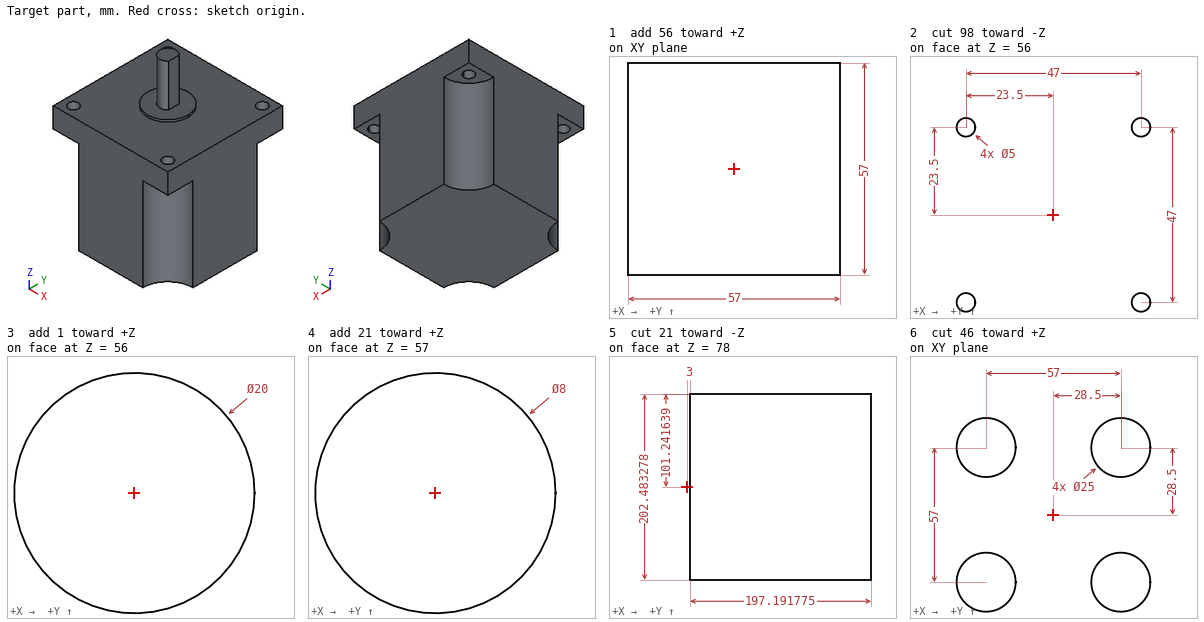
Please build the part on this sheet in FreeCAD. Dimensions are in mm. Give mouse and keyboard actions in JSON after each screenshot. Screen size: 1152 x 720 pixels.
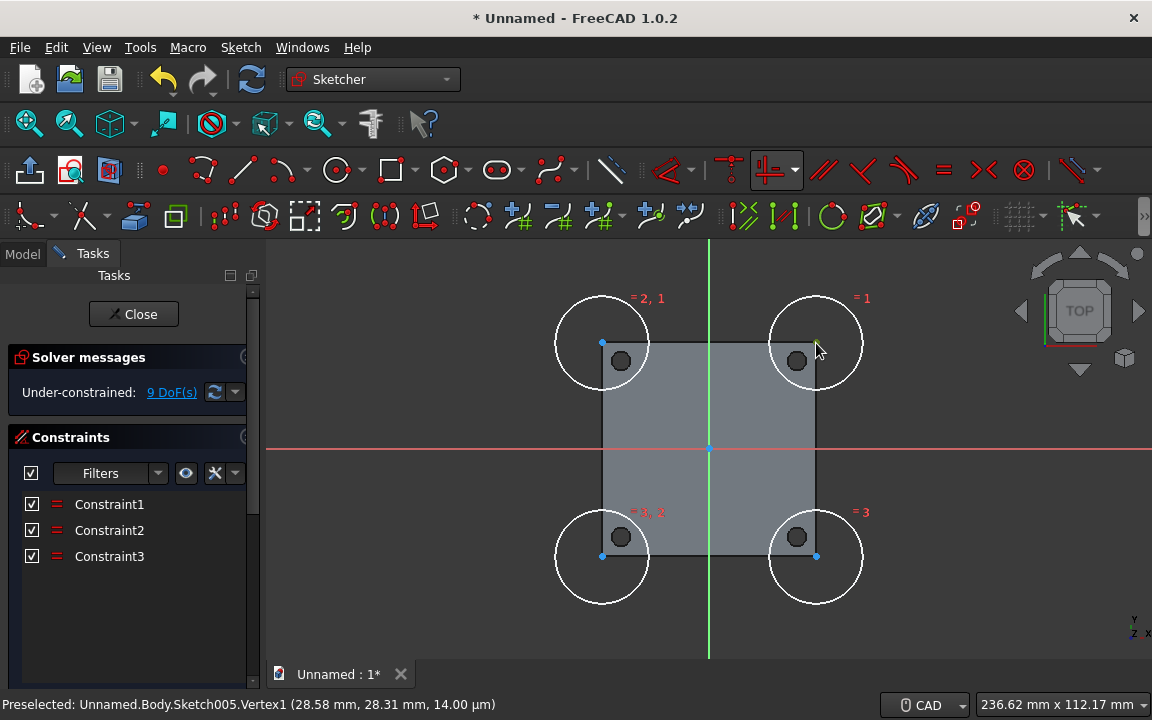
{"action": "left_click", "coordinate": [602, 343]}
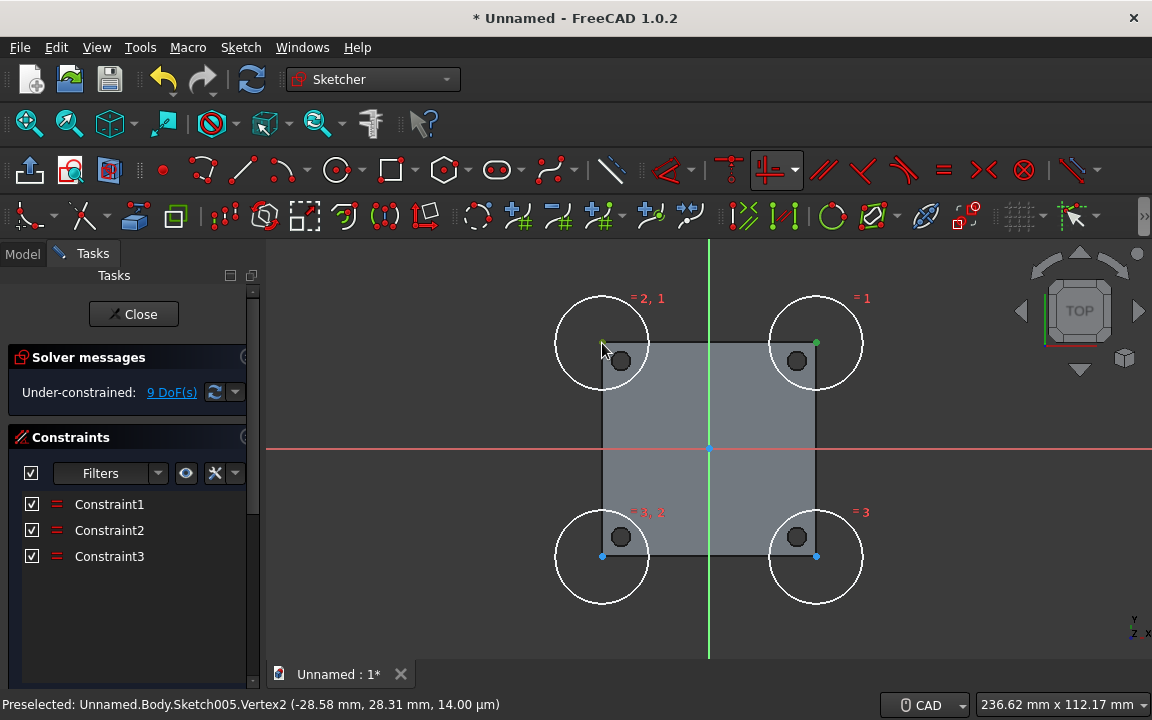
{"action": "left_click", "coordinate": [798, 170]}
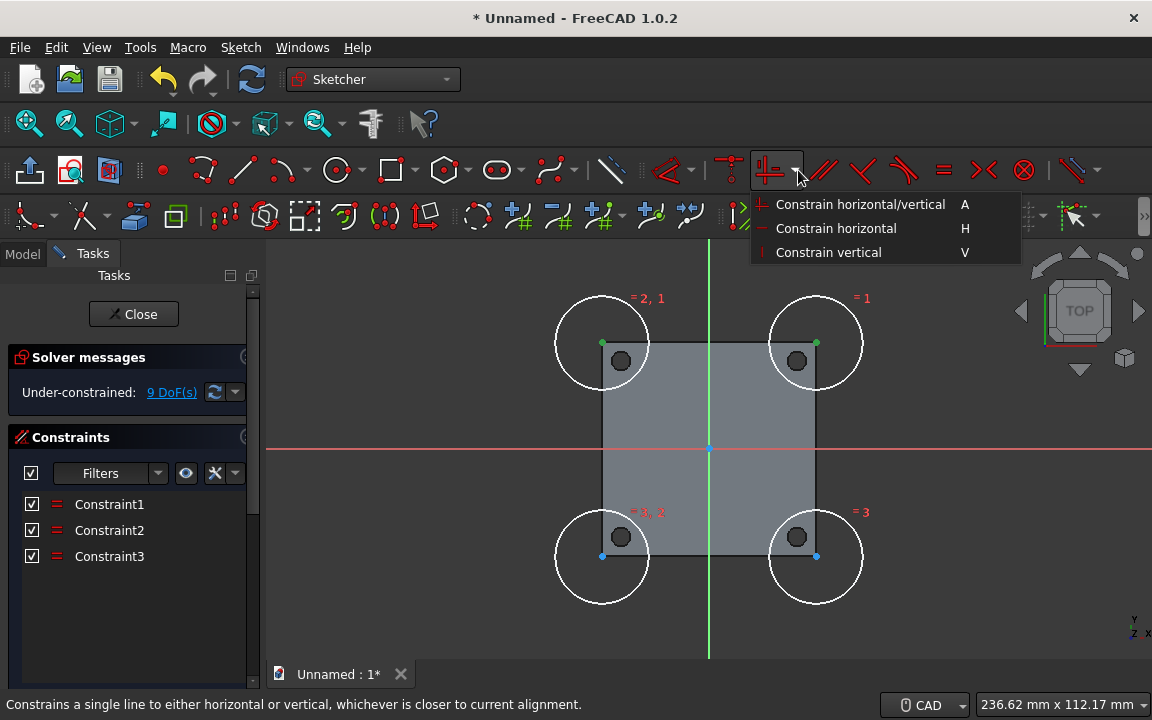
{"action": "left_click", "coordinate": [886, 228]}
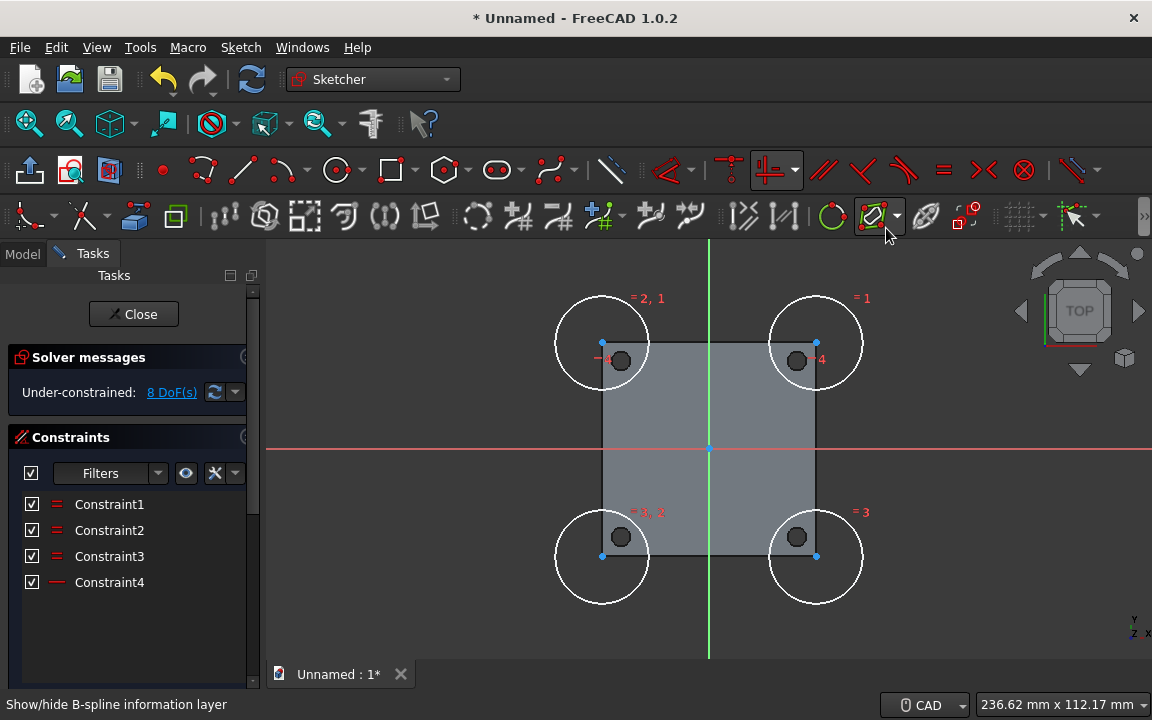
{"action": "left_click", "coordinate": [602, 343]}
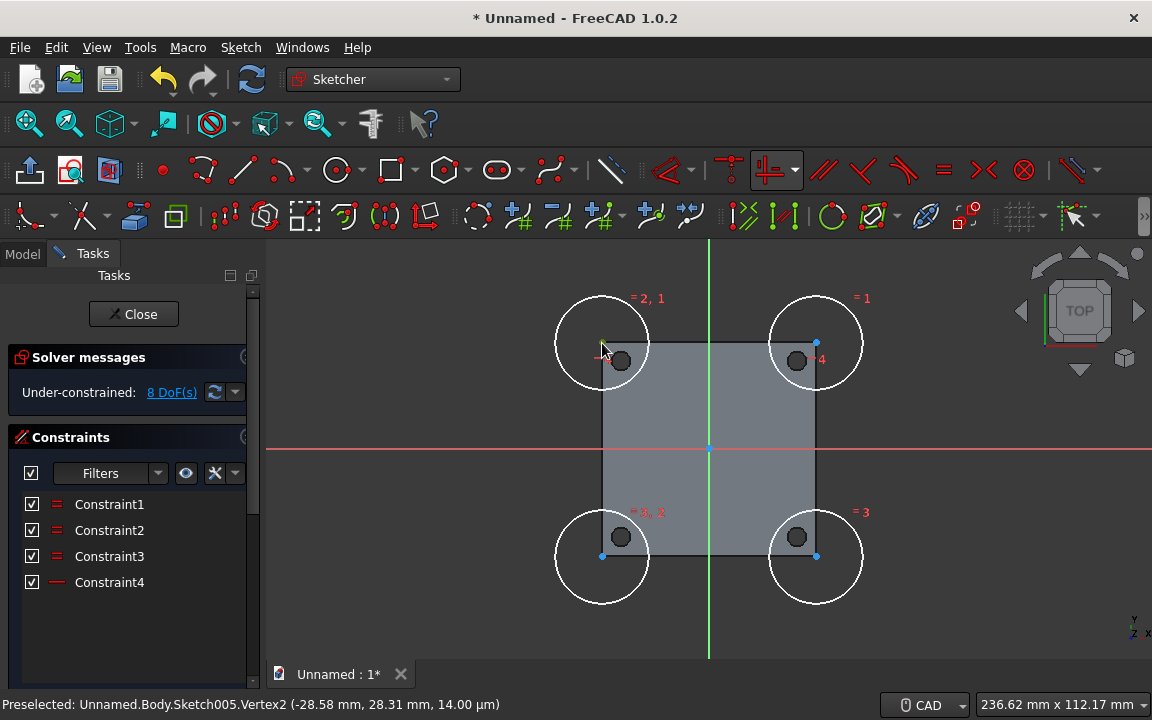
{"action": "left_click", "coordinate": [602, 557]}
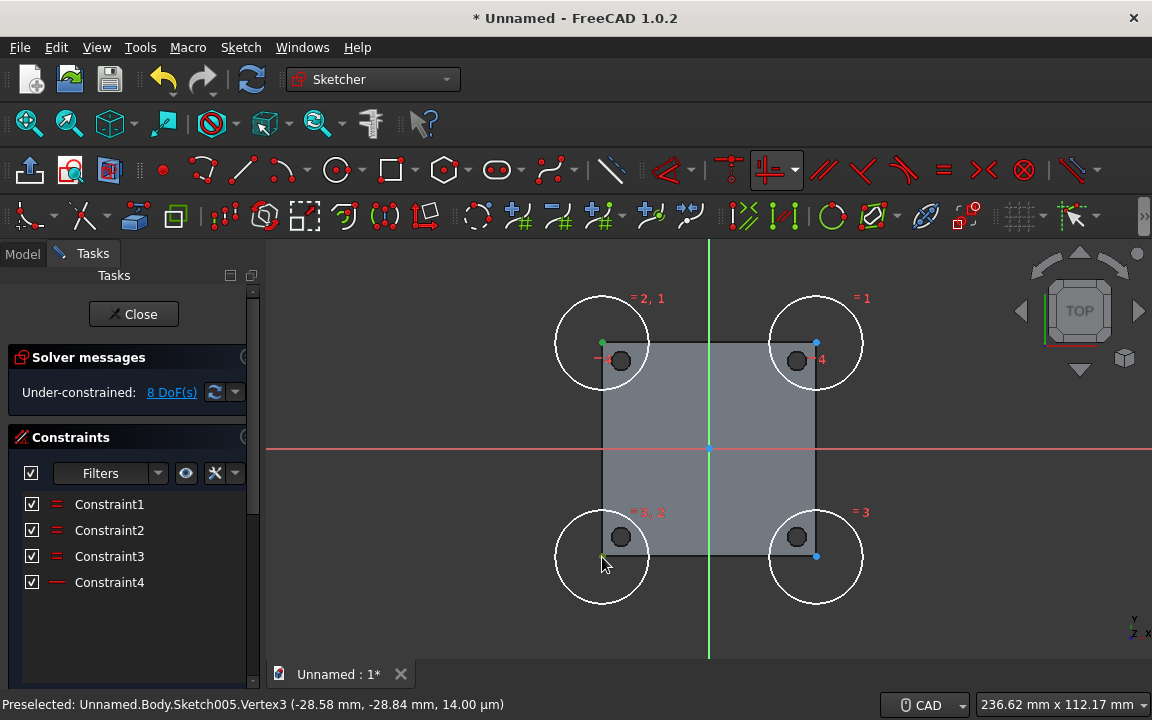
{"action": "left_click", "coordinate": [798, 170]}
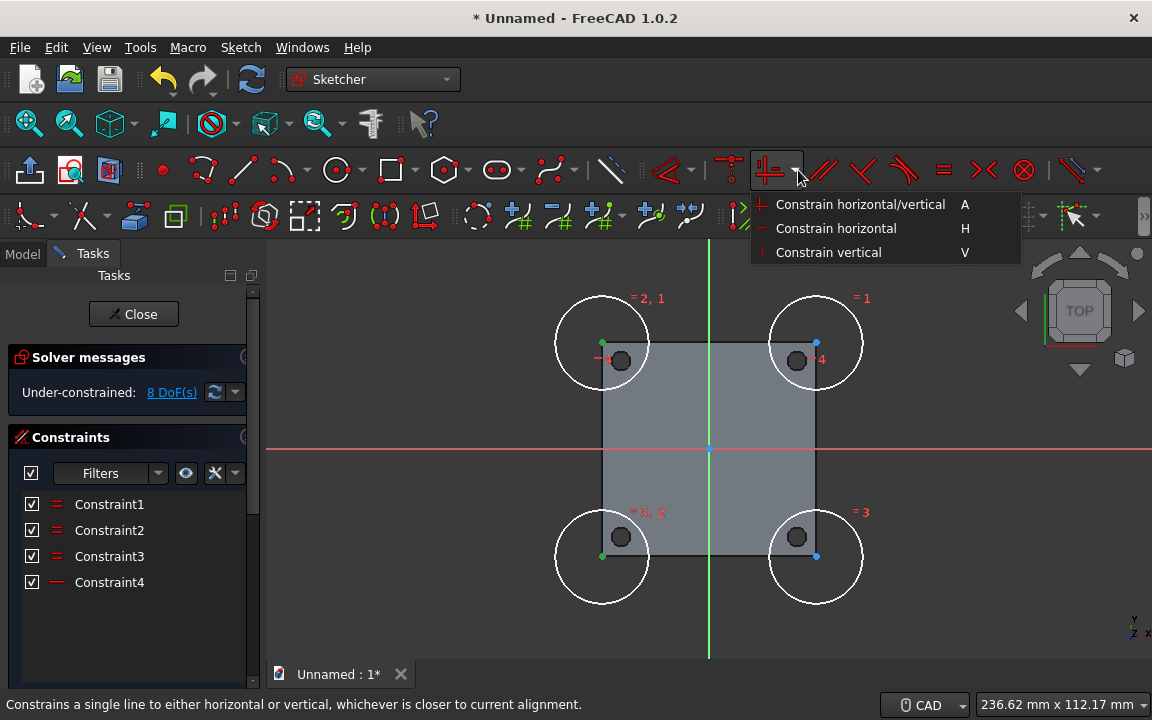
{"action": "left_click", "coordinate": [886, 252]}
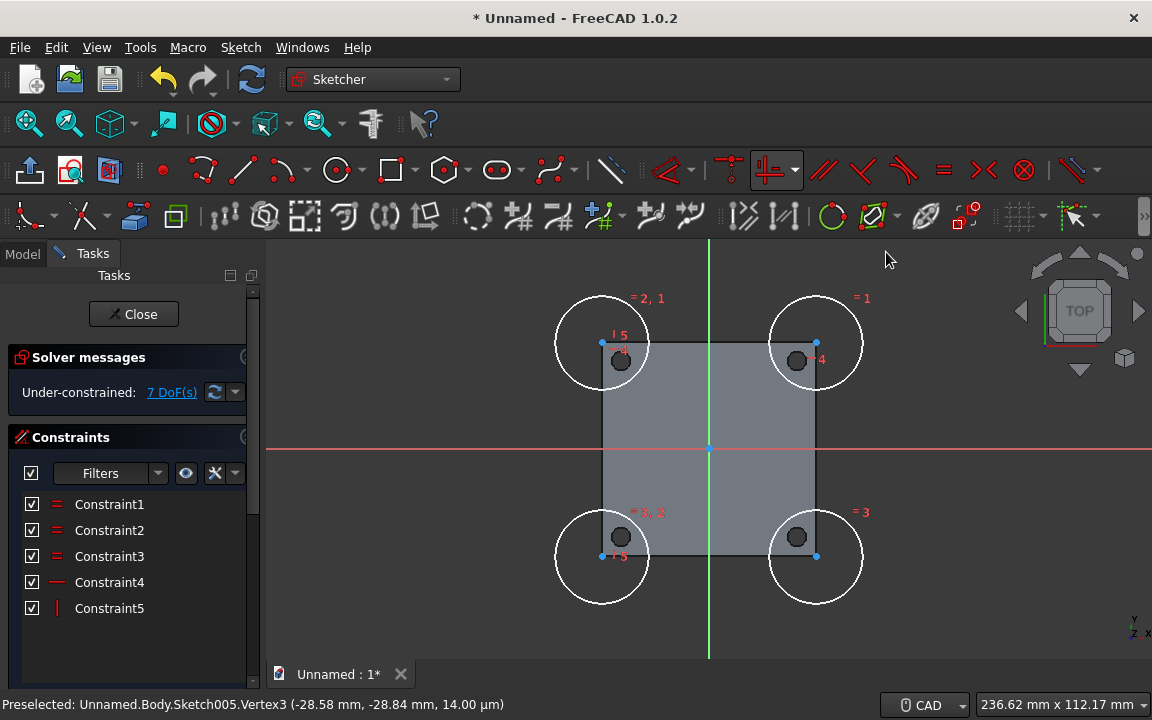
{"action": "left_click", "coordinate": [816, 343]}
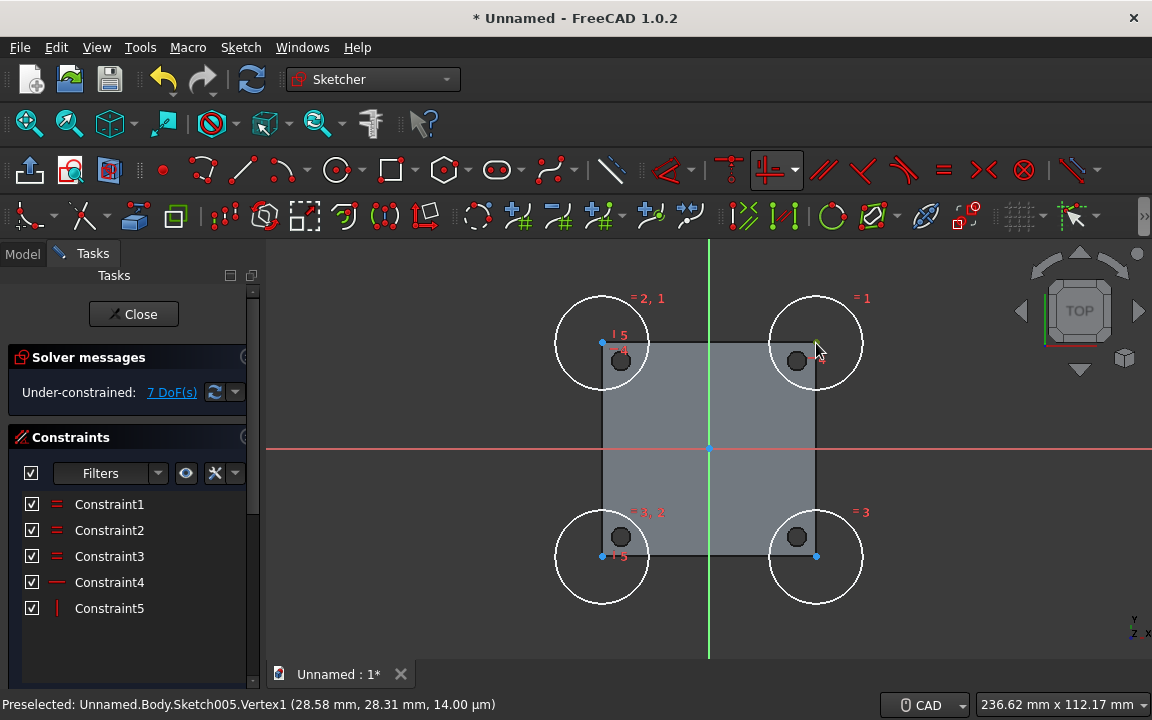
{"action": "left_click", "coordinate": [816, 557]}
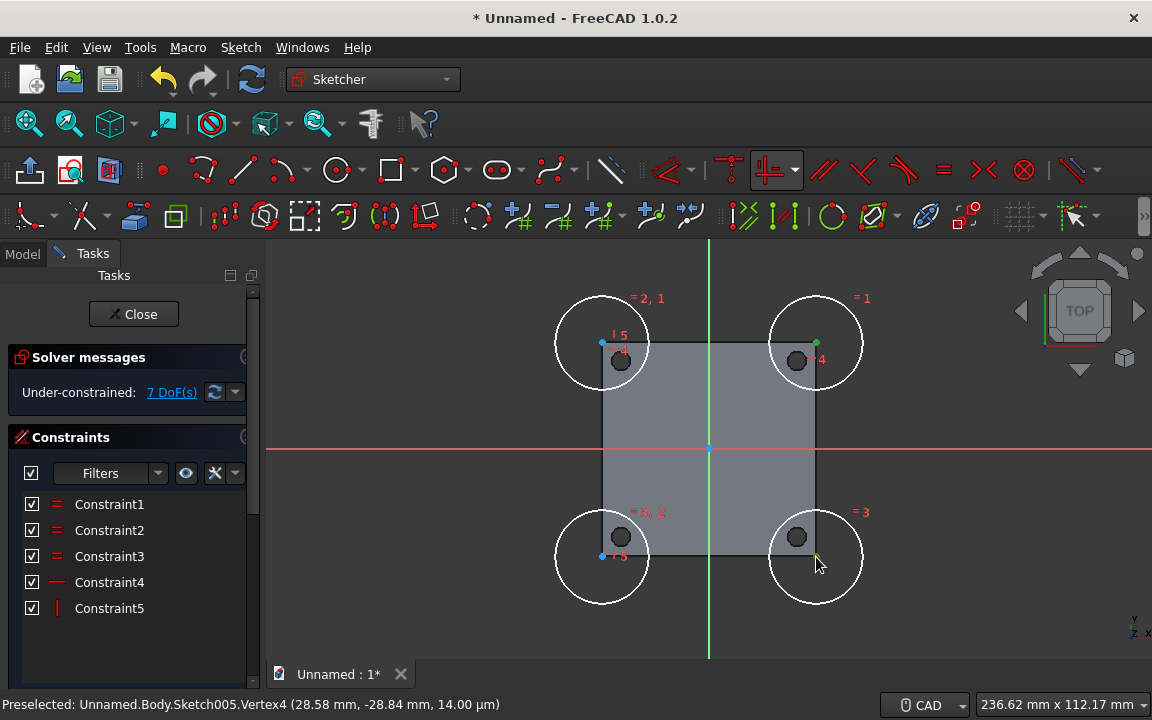
{"action": "key", "text": "v"}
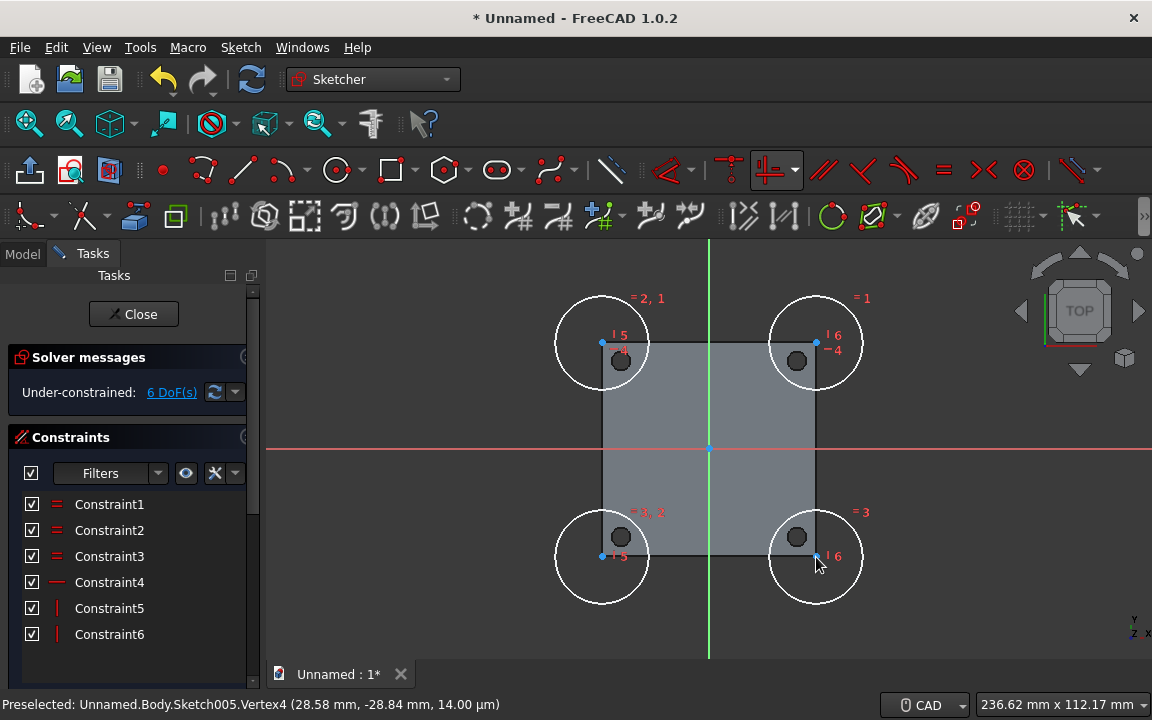
{"action": "left_click", "coordinate": [602, 557]}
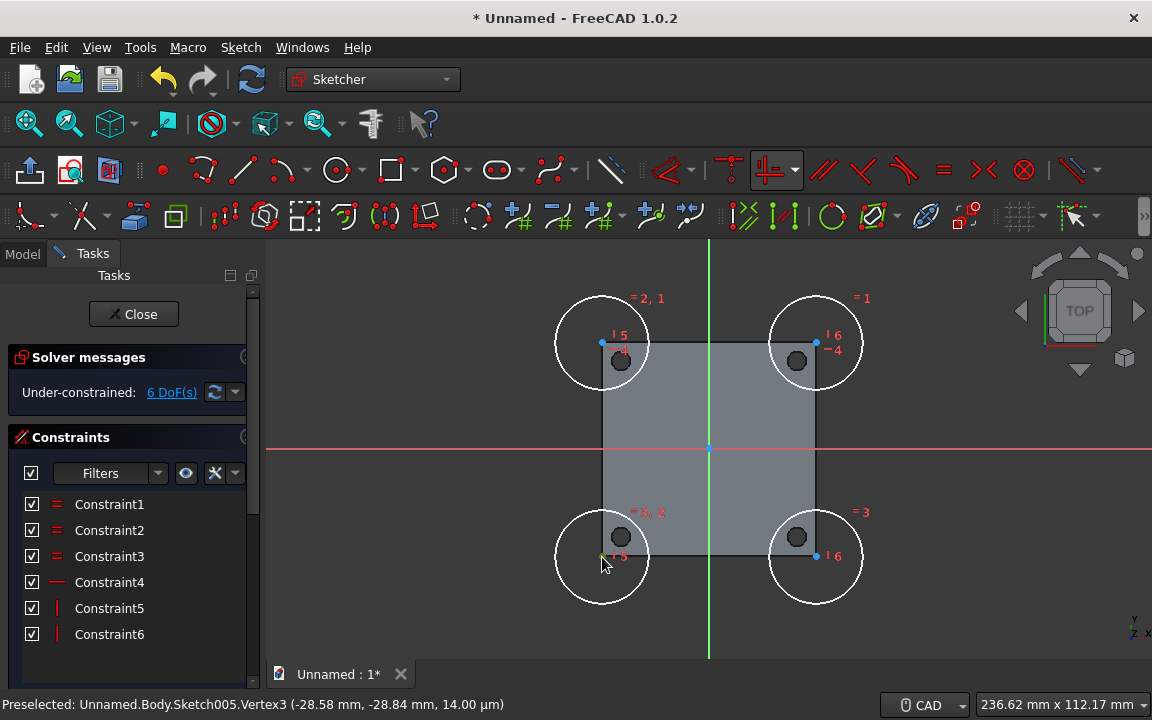
{"action": "left_click", "coordinate": [816, 557]}